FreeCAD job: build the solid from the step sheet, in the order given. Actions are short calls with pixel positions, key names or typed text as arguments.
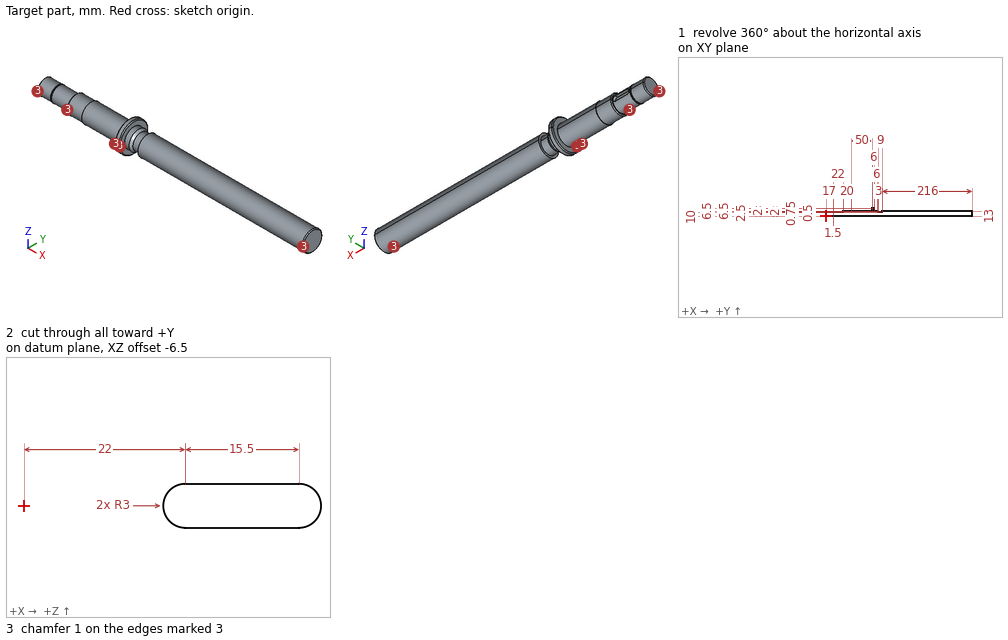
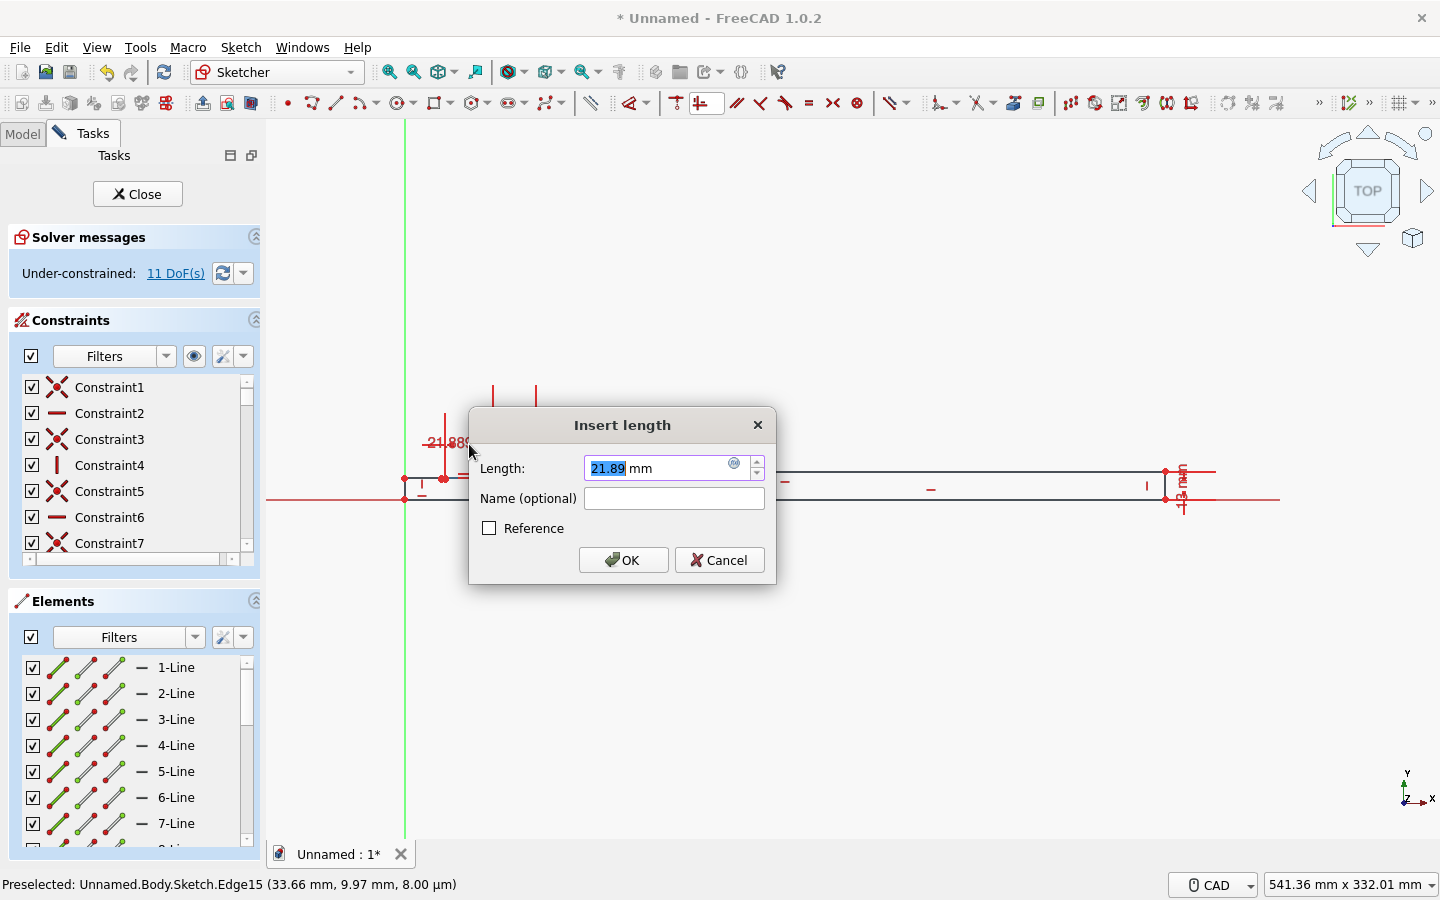
text(22)
key(Return)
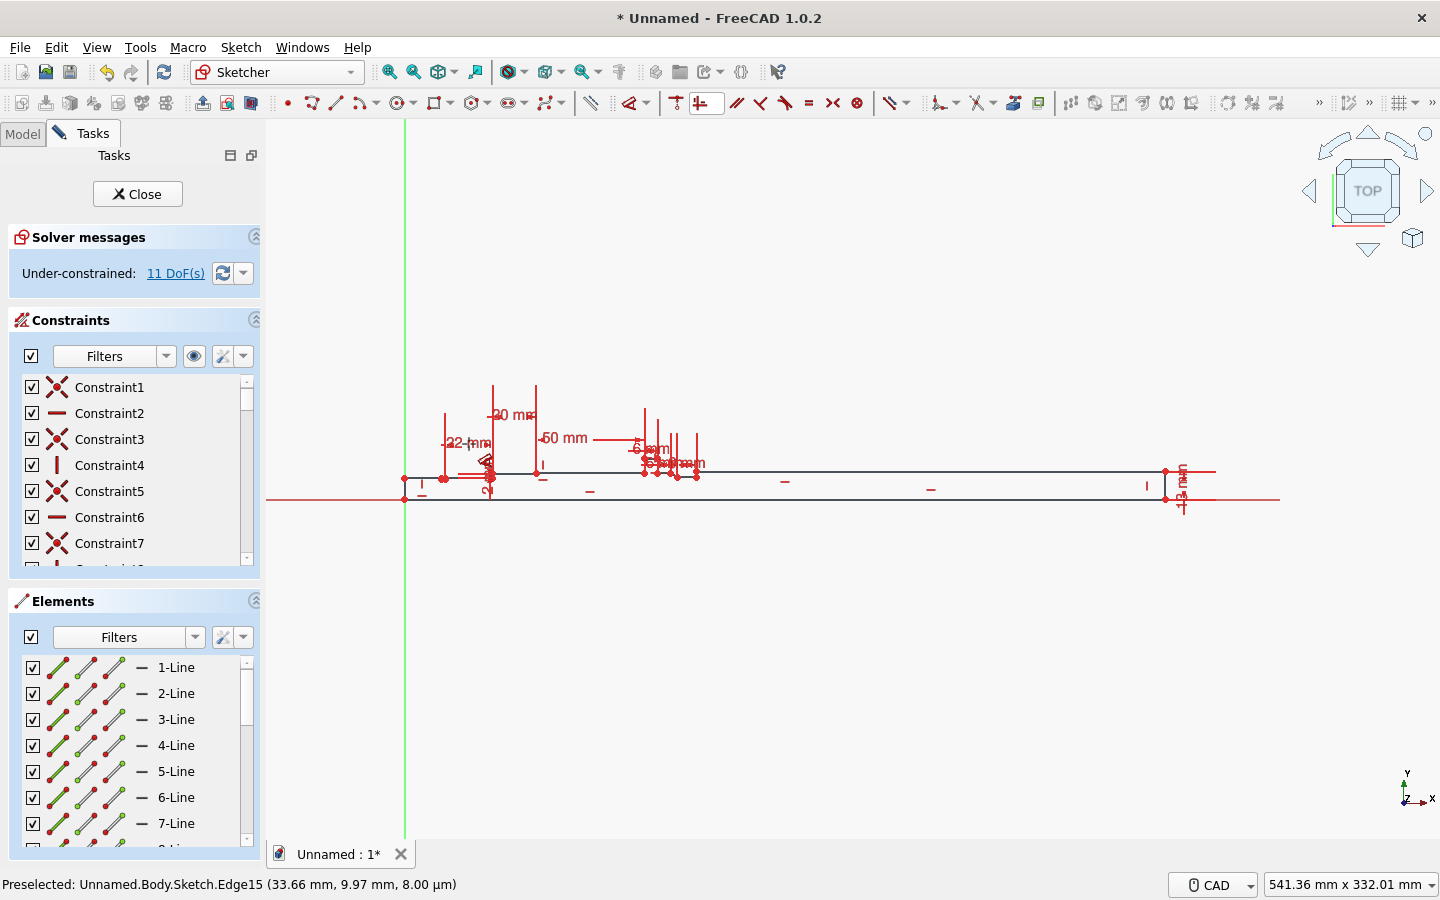
scroll(431, 478, up, 2)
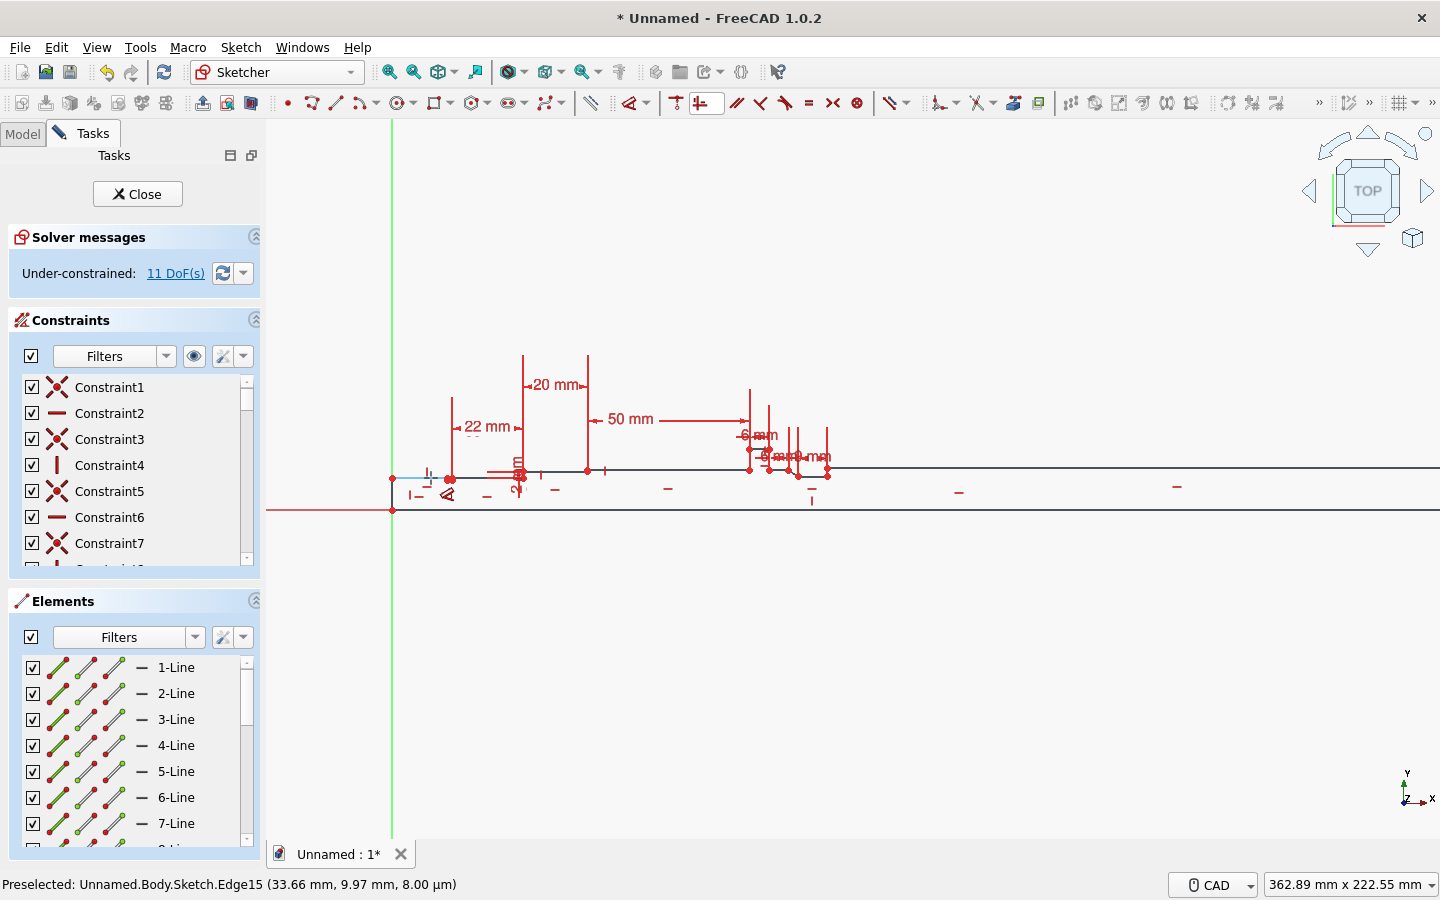
click(431, 478)
click(407, 444)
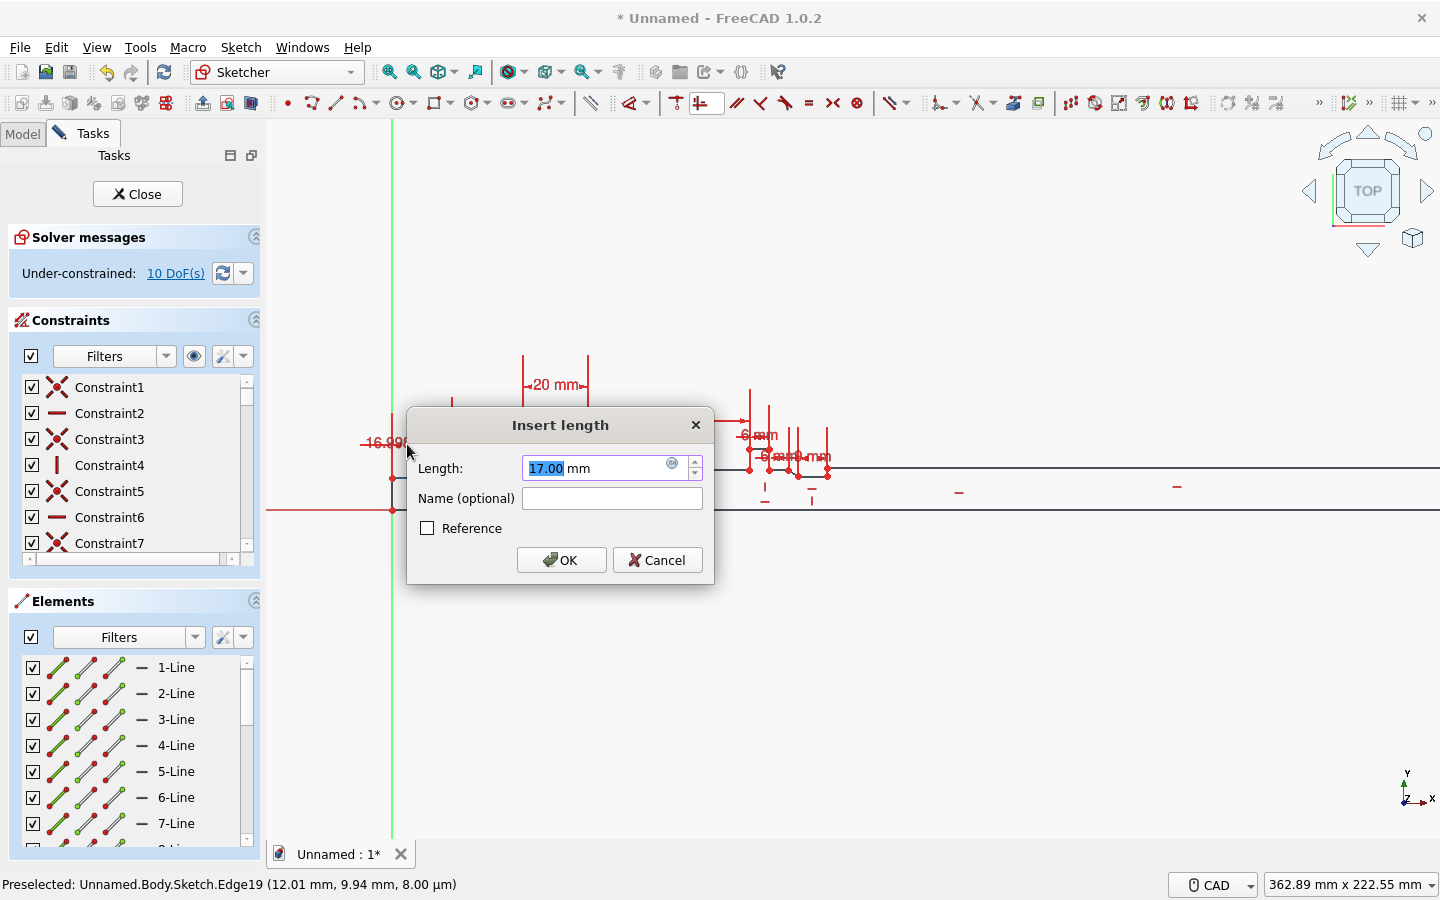
text(17)
key(Return)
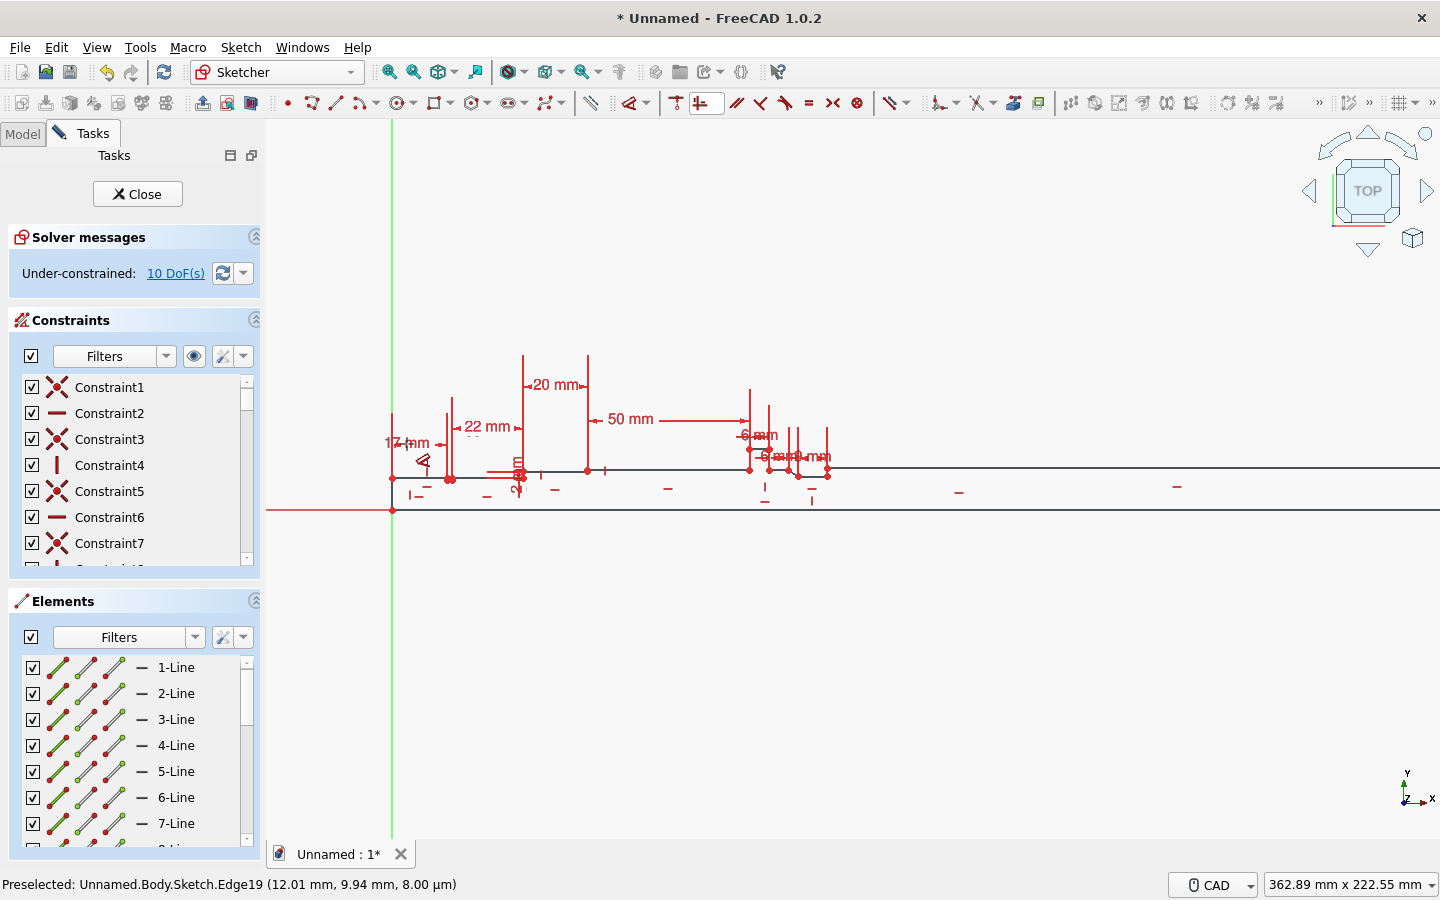
scroll(392, 488, up, 2)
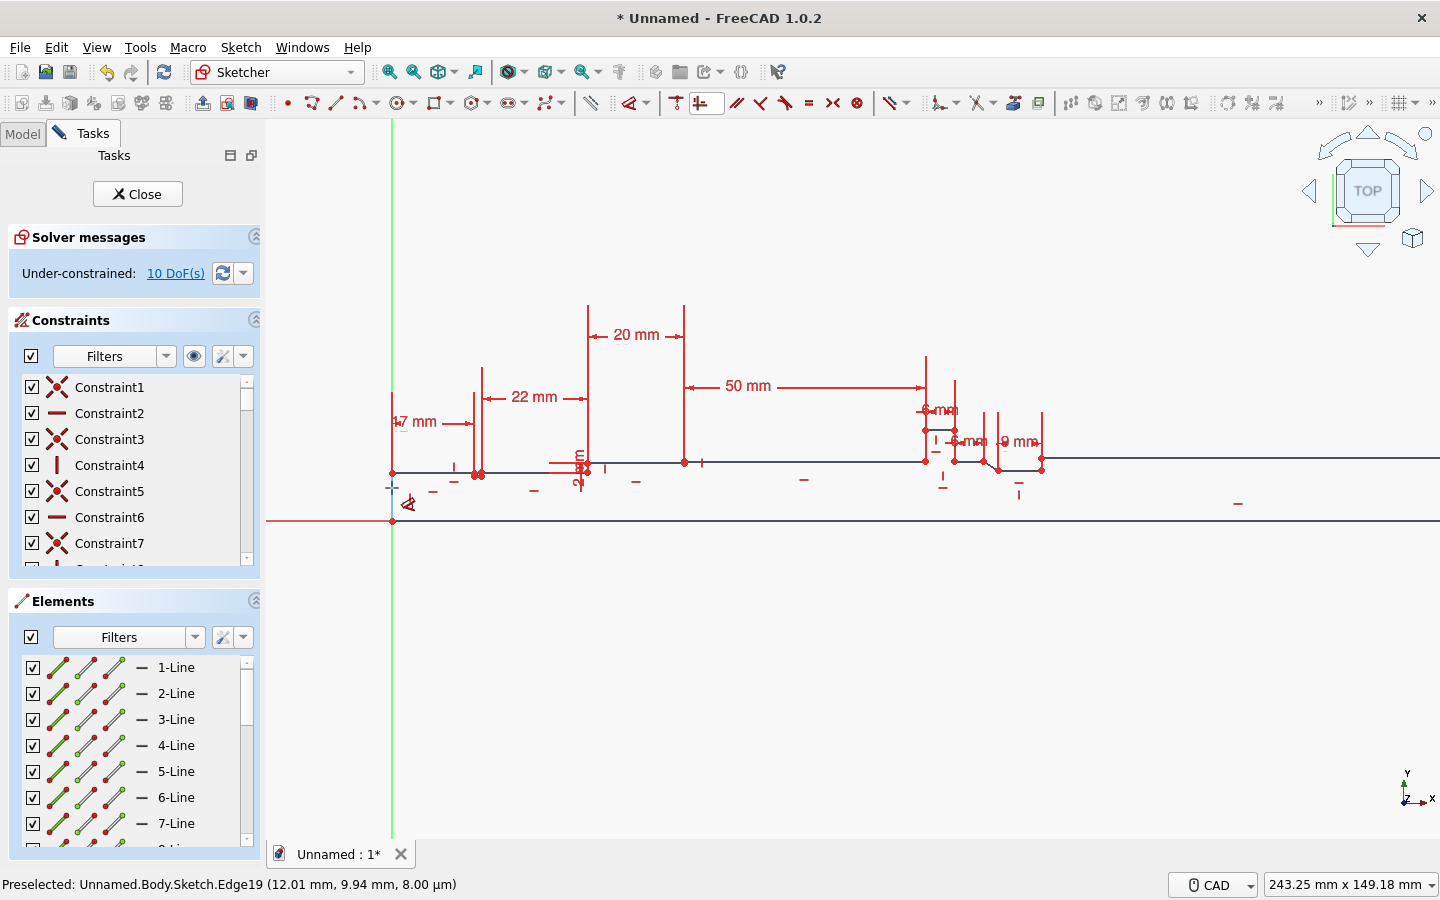
click(392, 487)
click(358, 497)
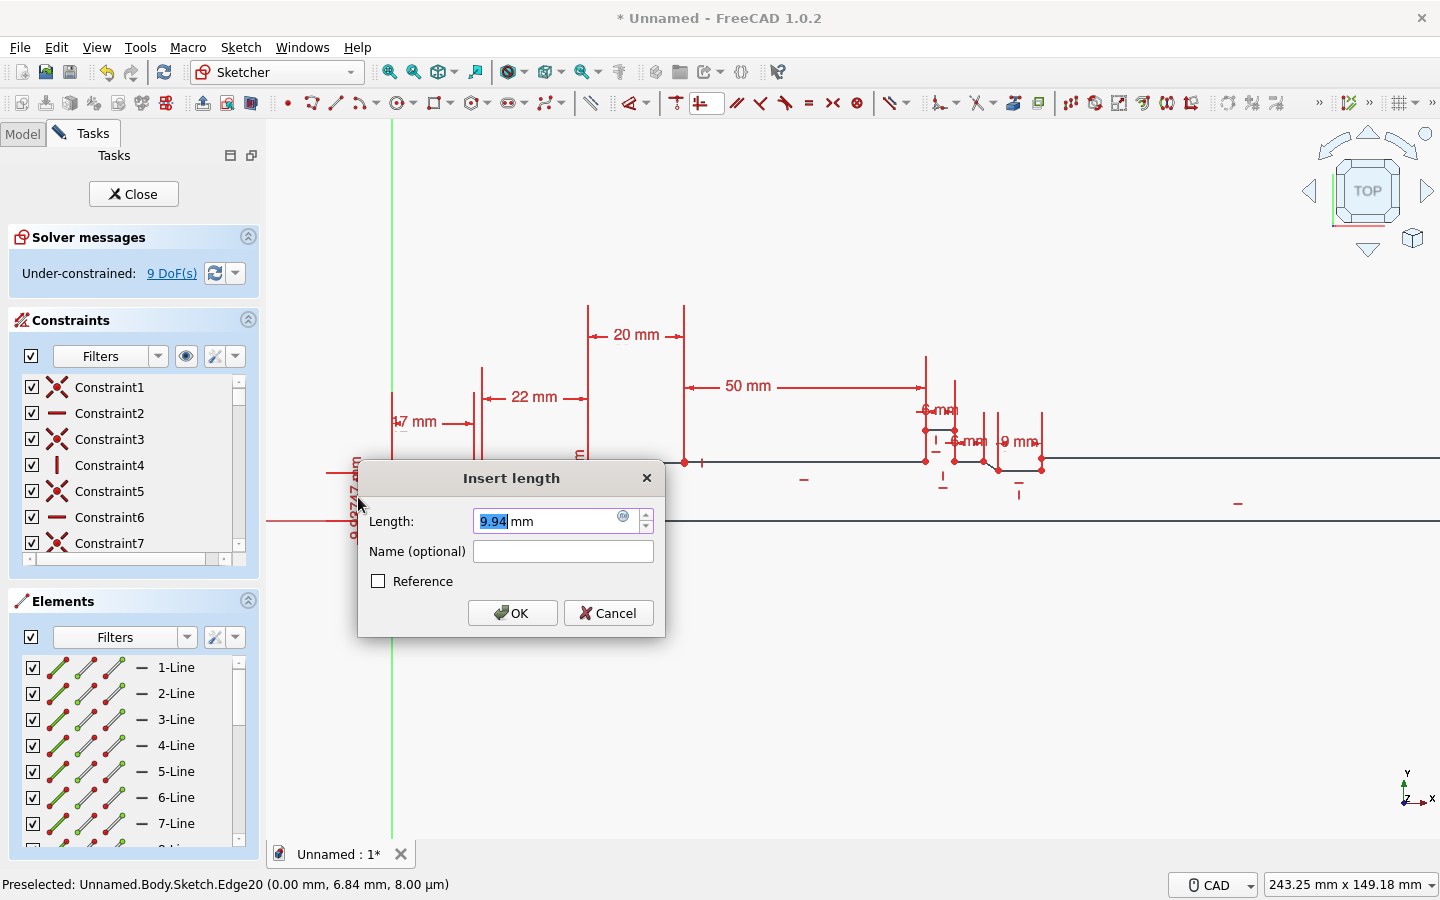
text(10)
key(Return)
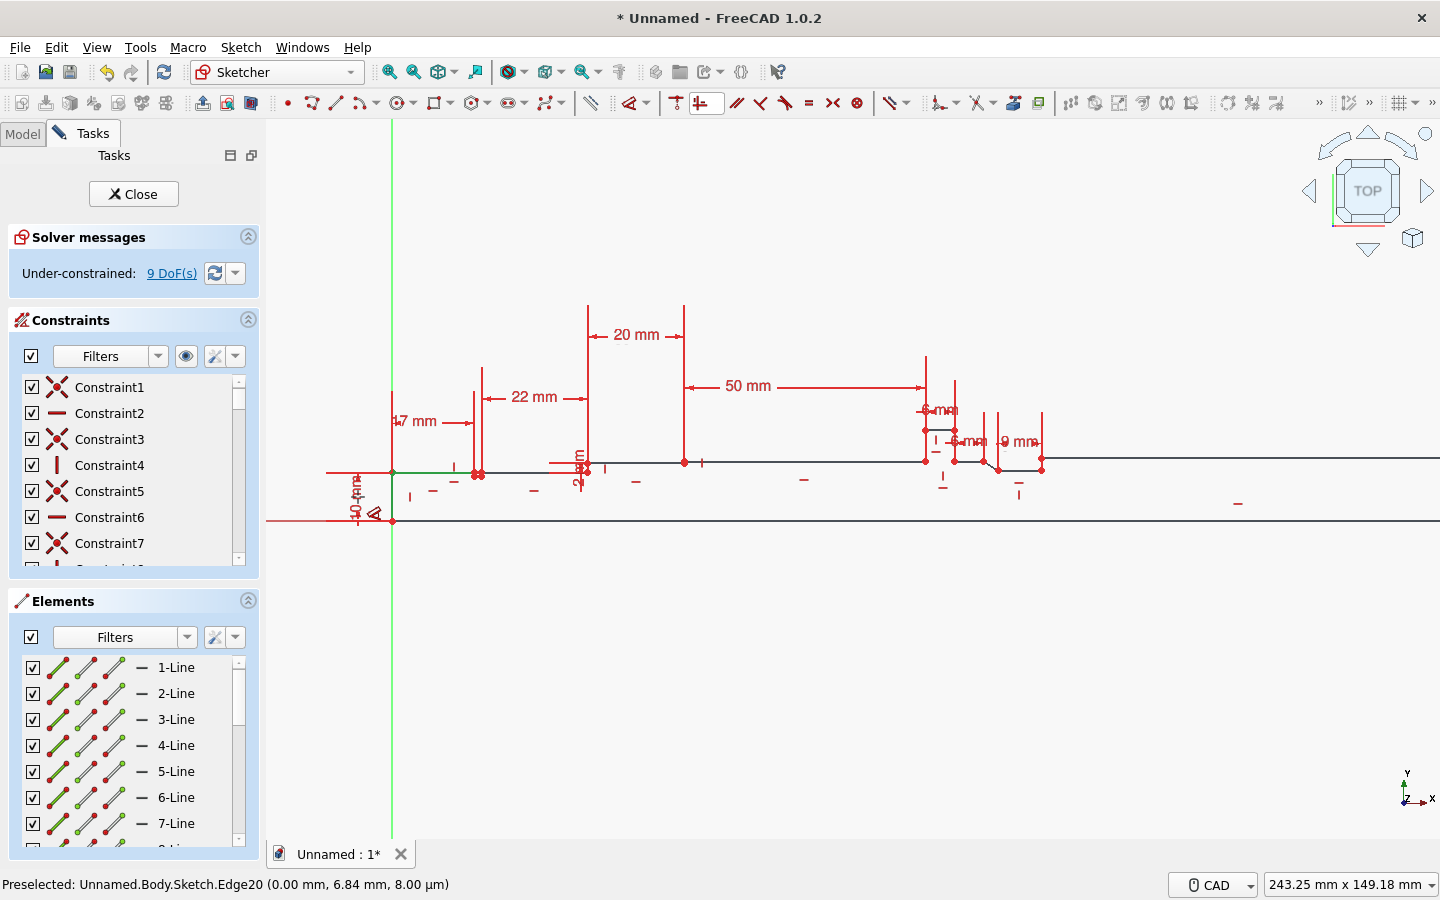
scroll(991, 466, up, 6)